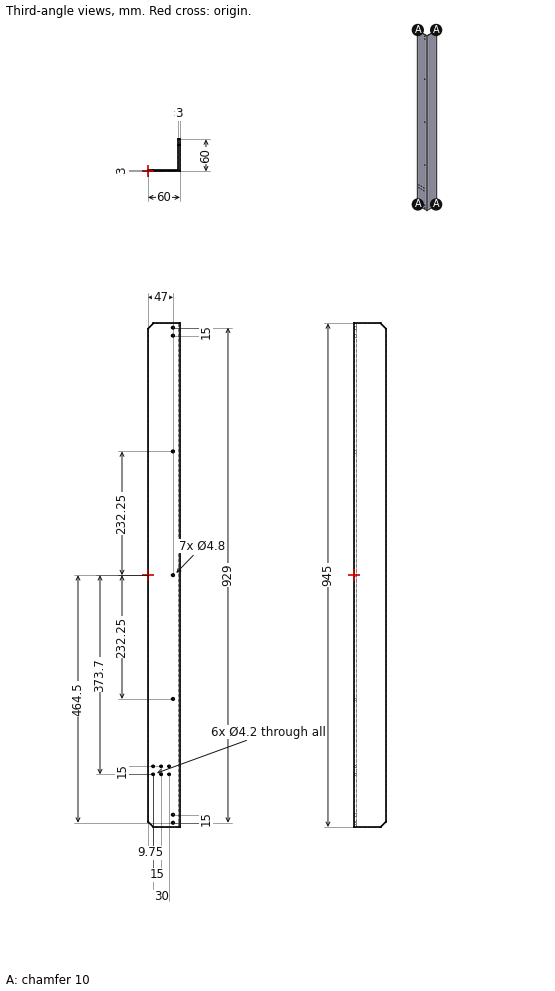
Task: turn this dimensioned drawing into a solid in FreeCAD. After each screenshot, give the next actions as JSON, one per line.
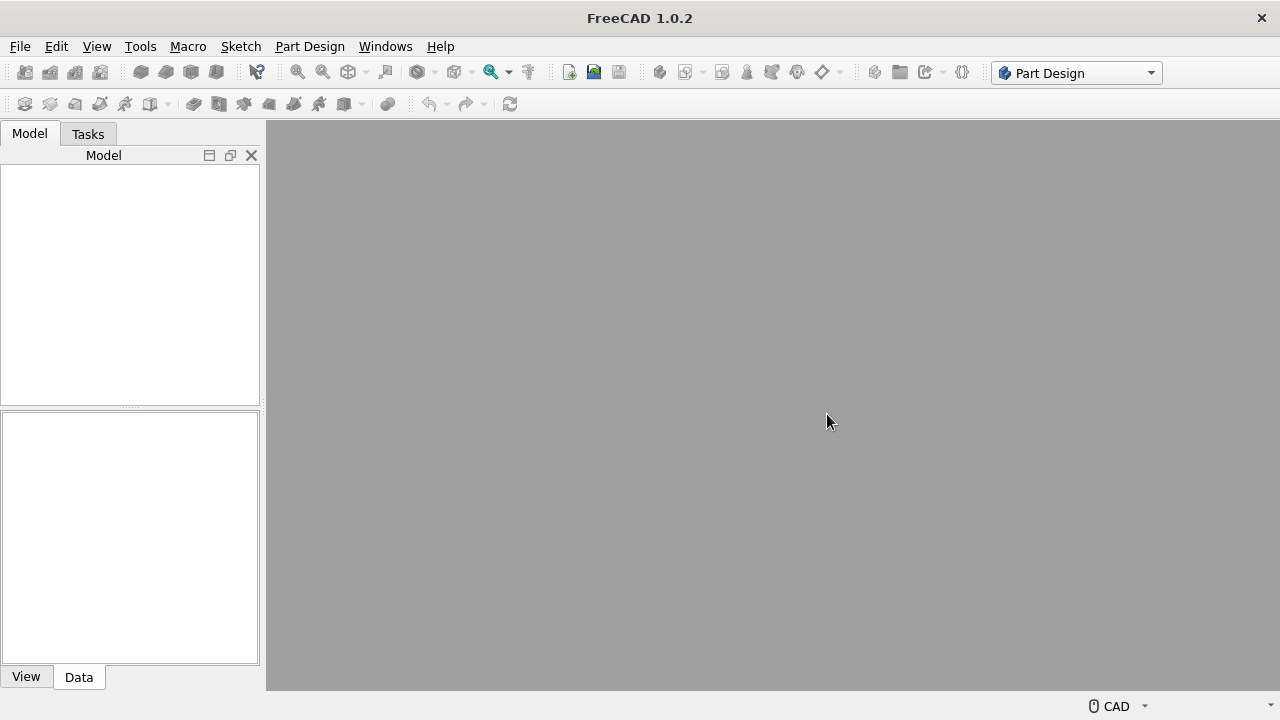
{"action": "left_click", "coordinate": [569, 72]}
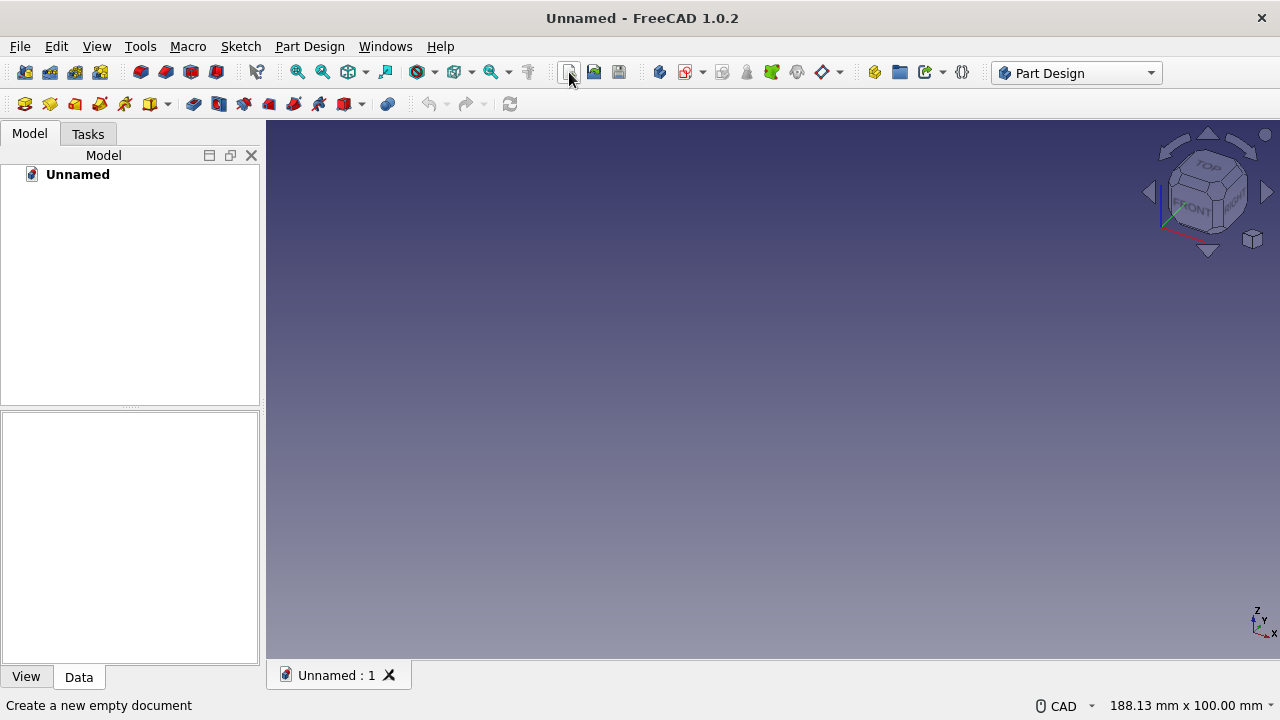
{"action": "left_click", "coordinate": [684, 72]}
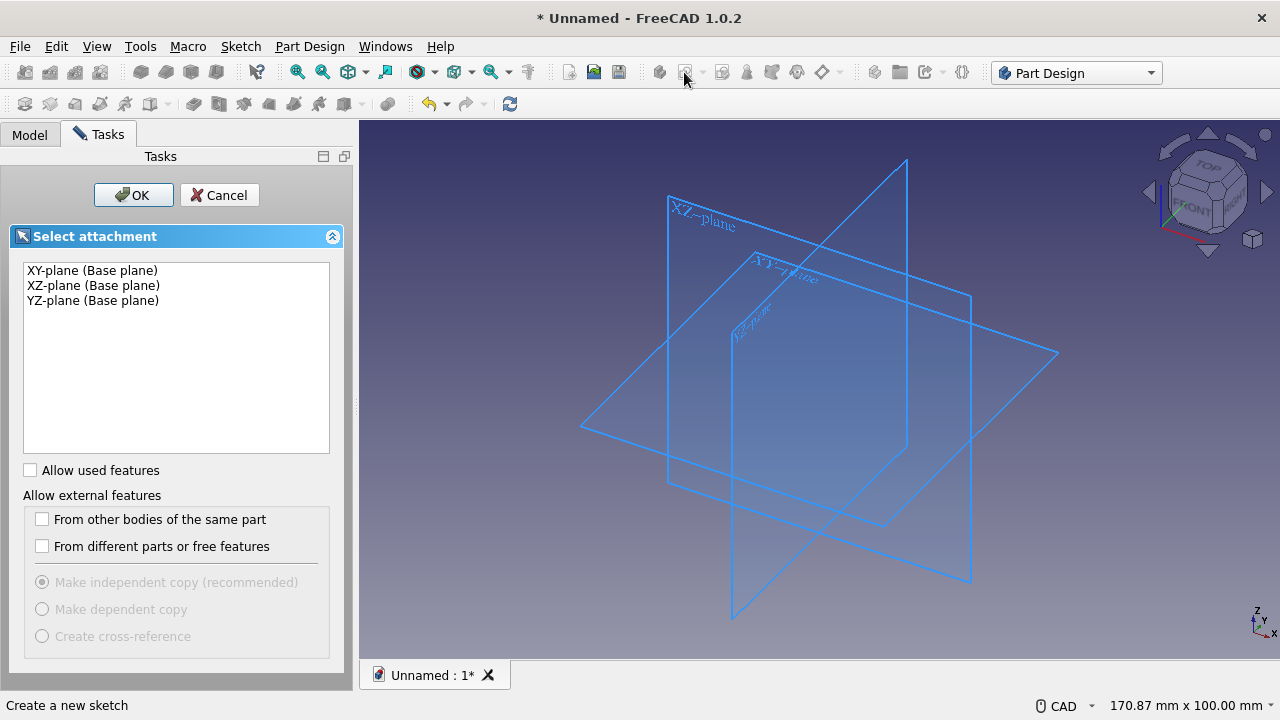
{"action": "left_click", "coordinate": [84, 270]}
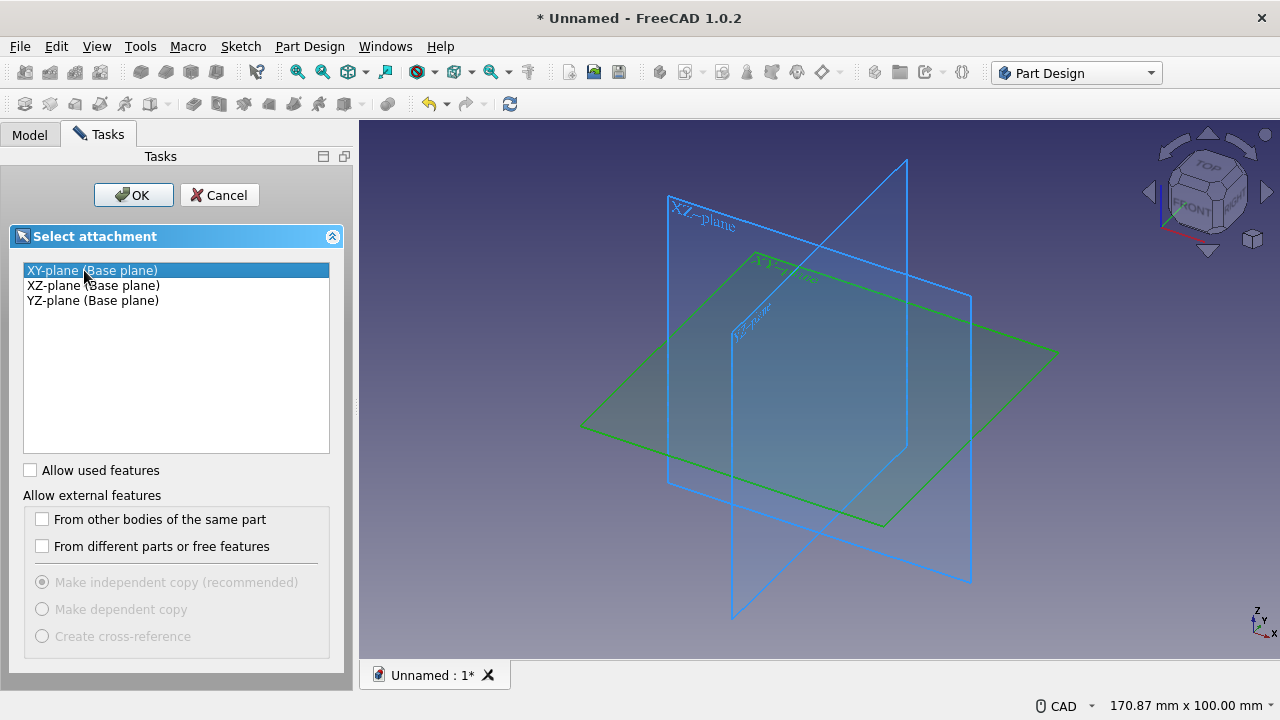
{"action": "left_click", "coordinate": [134, 195]}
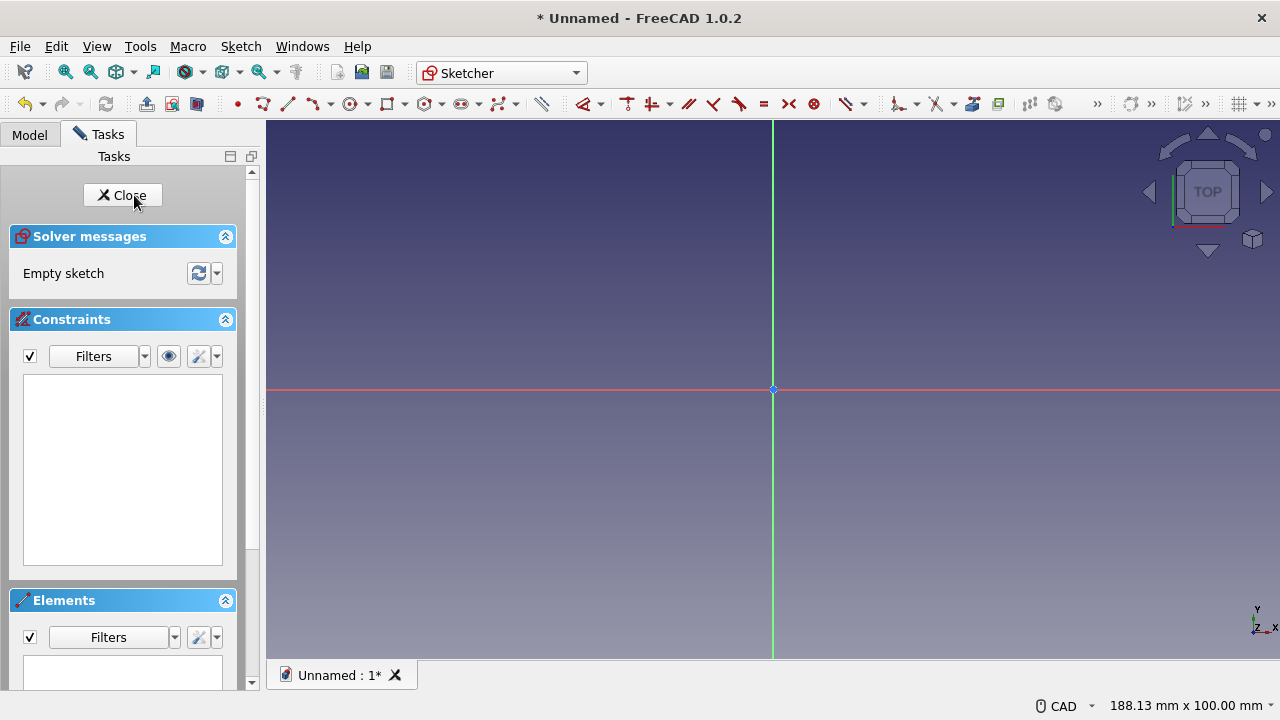
{"action": "scroll", "coordinate": [294, 631], "scroll_direction": "down", "scroll_amount": 2}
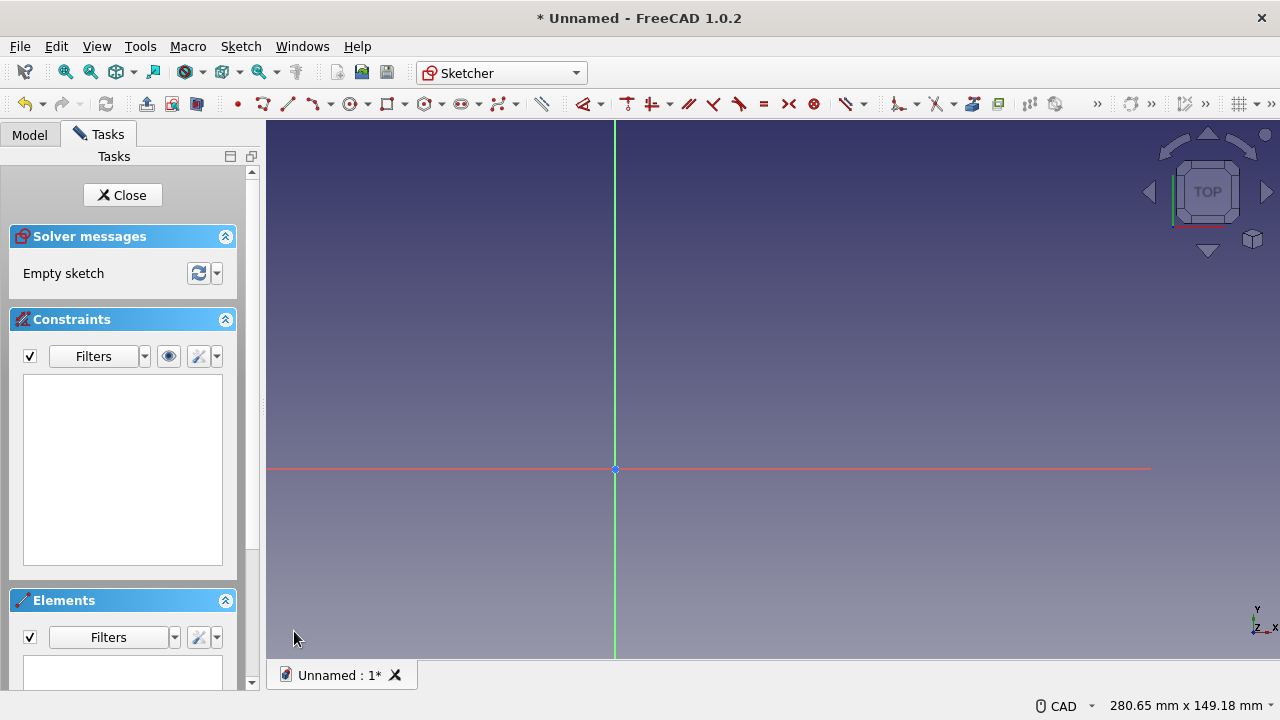
{"action": "scroll", "coordinate": [762, 303], "scroll_direction": "up", "scroll_amount": 2}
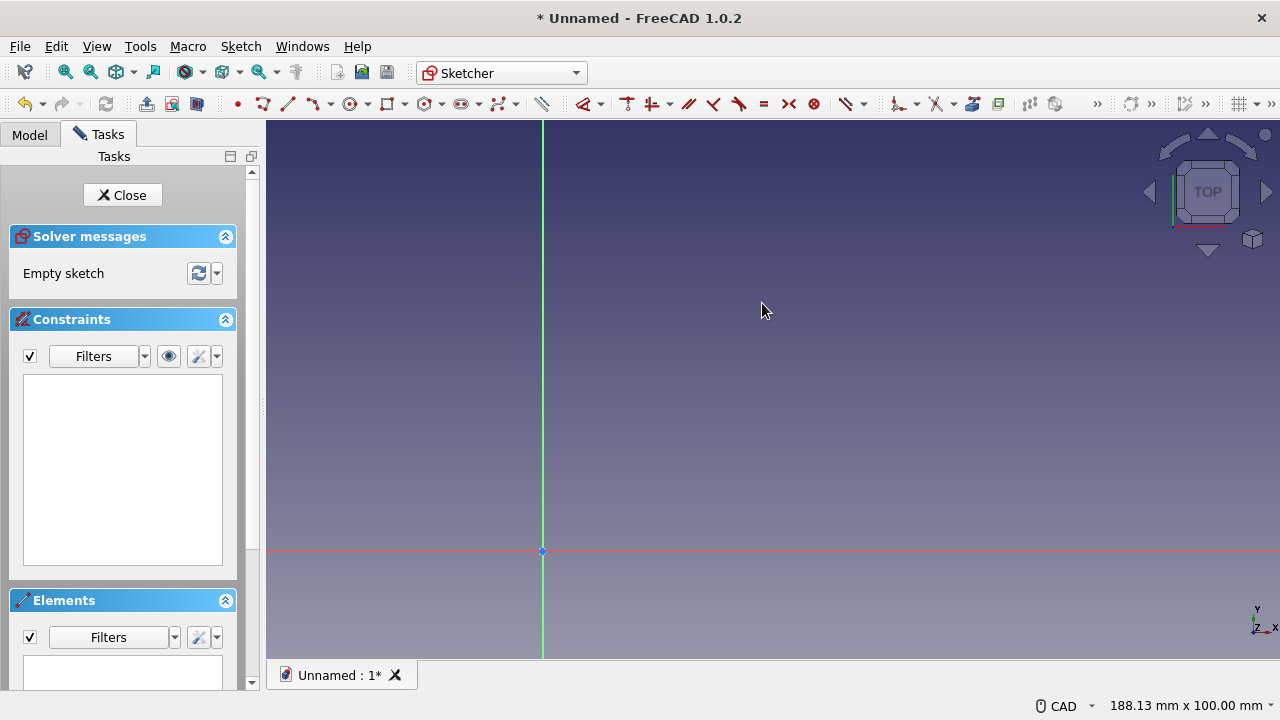
{"action": "left_click", "coordinate": [263, 104]}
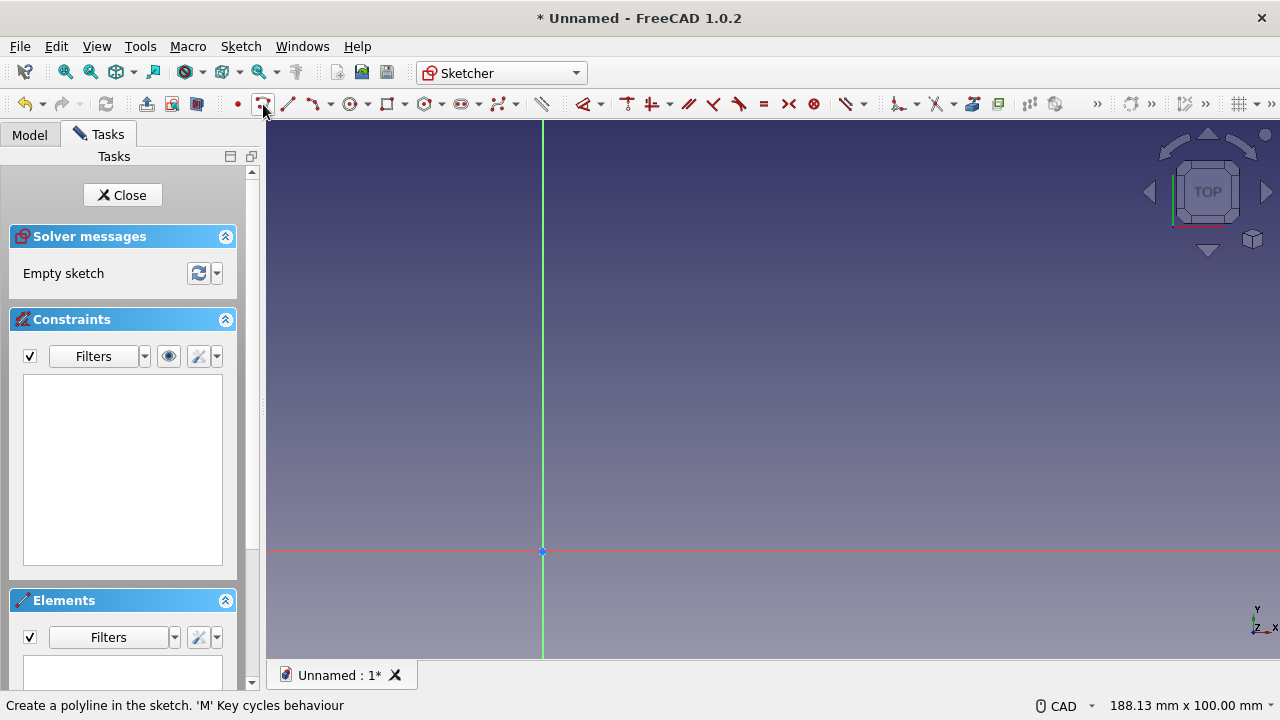
{"action": "left_click", "coordinate": [543, 551]}
{"action": "left_click", "coordinate": [866, 542]}
{"action": "left_click", "coordinate": [866, 228]}
{"action": "left_click", "coordinate": [850, 228]}
{"action": "left_click", "coordinate": [850, 535]}
{"action": "left_click", "coordinate": [552, 535]}
{"action": "left_click", "coordinate": [543, 551]}
{"action": "key", "text": "Escape"}
{"action": "key", "text": "Escape"}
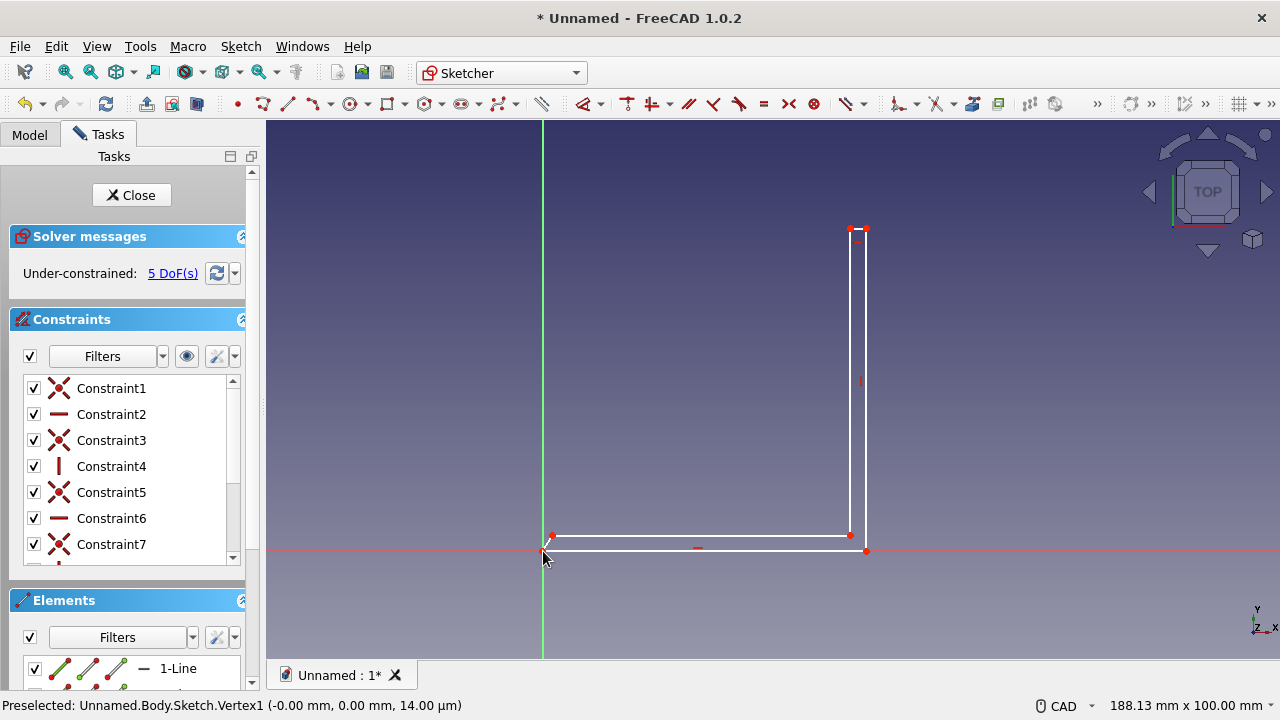
{"action": "scroll", "coordinate": [546, 545], "scroll_direction": "up", "scroll_amount": 5}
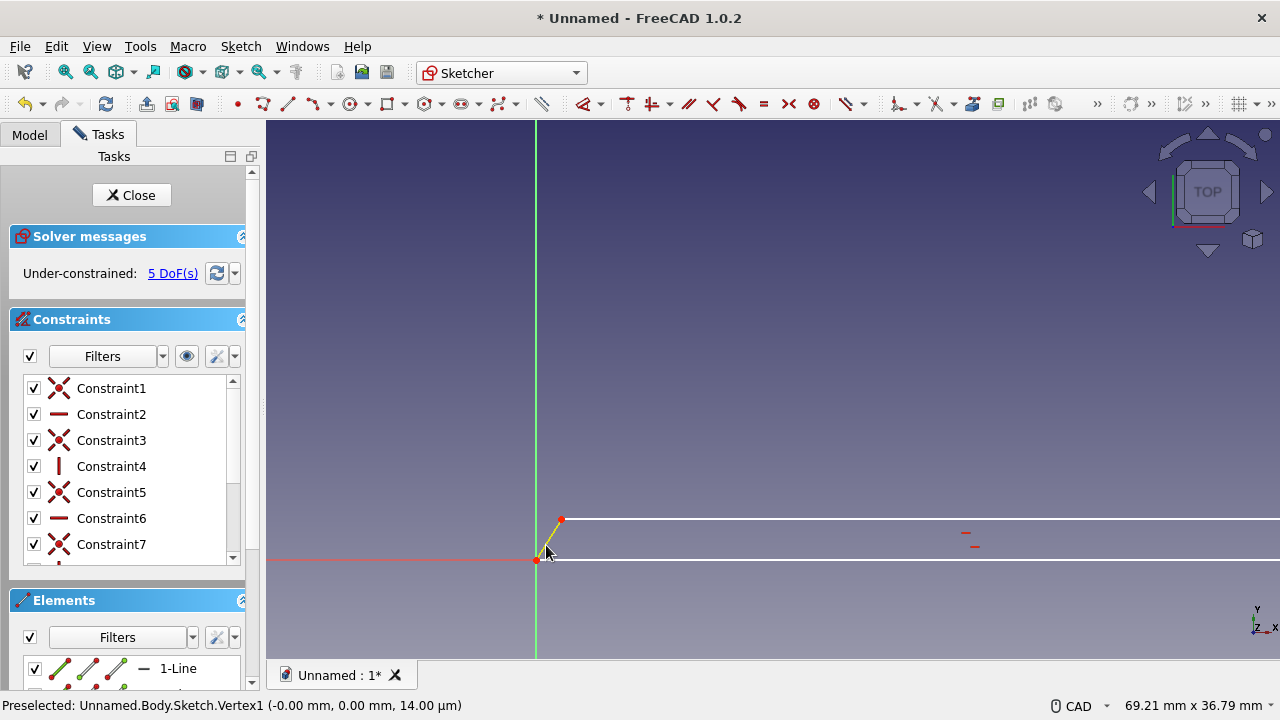
{"action": "left_click", "coordinate": [547, 544]}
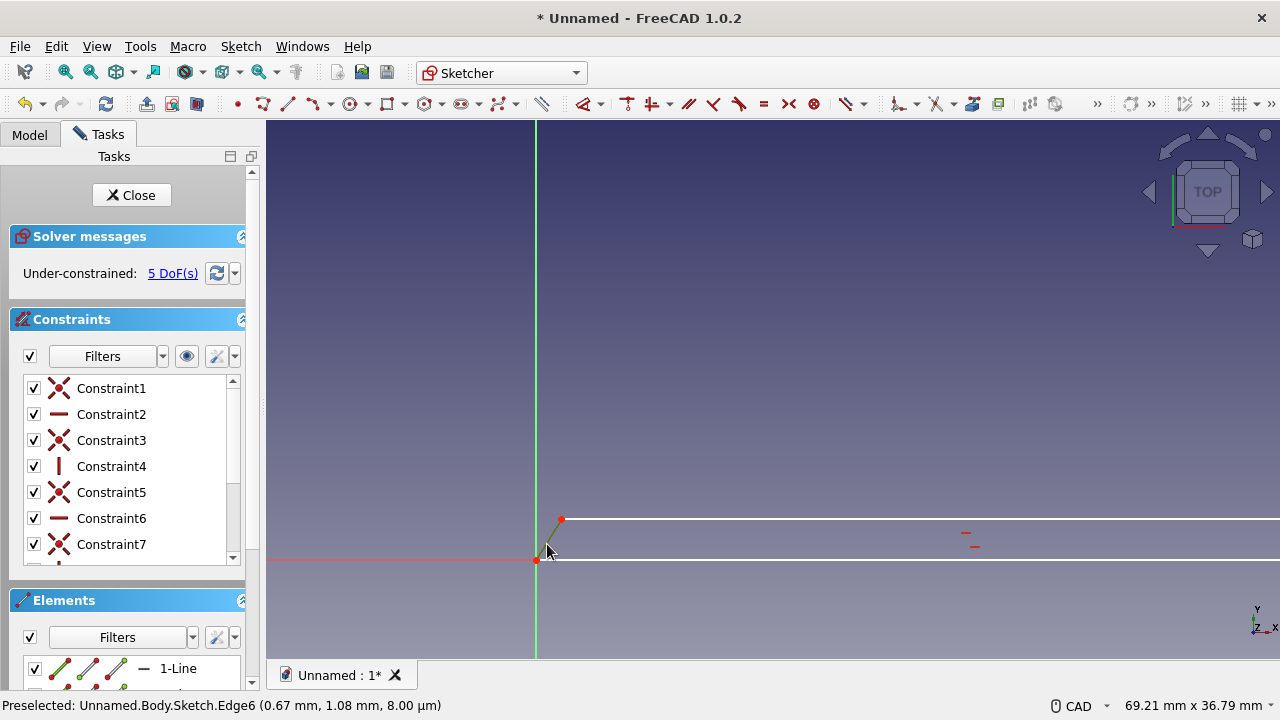
{"action": "key", "text": "v"}